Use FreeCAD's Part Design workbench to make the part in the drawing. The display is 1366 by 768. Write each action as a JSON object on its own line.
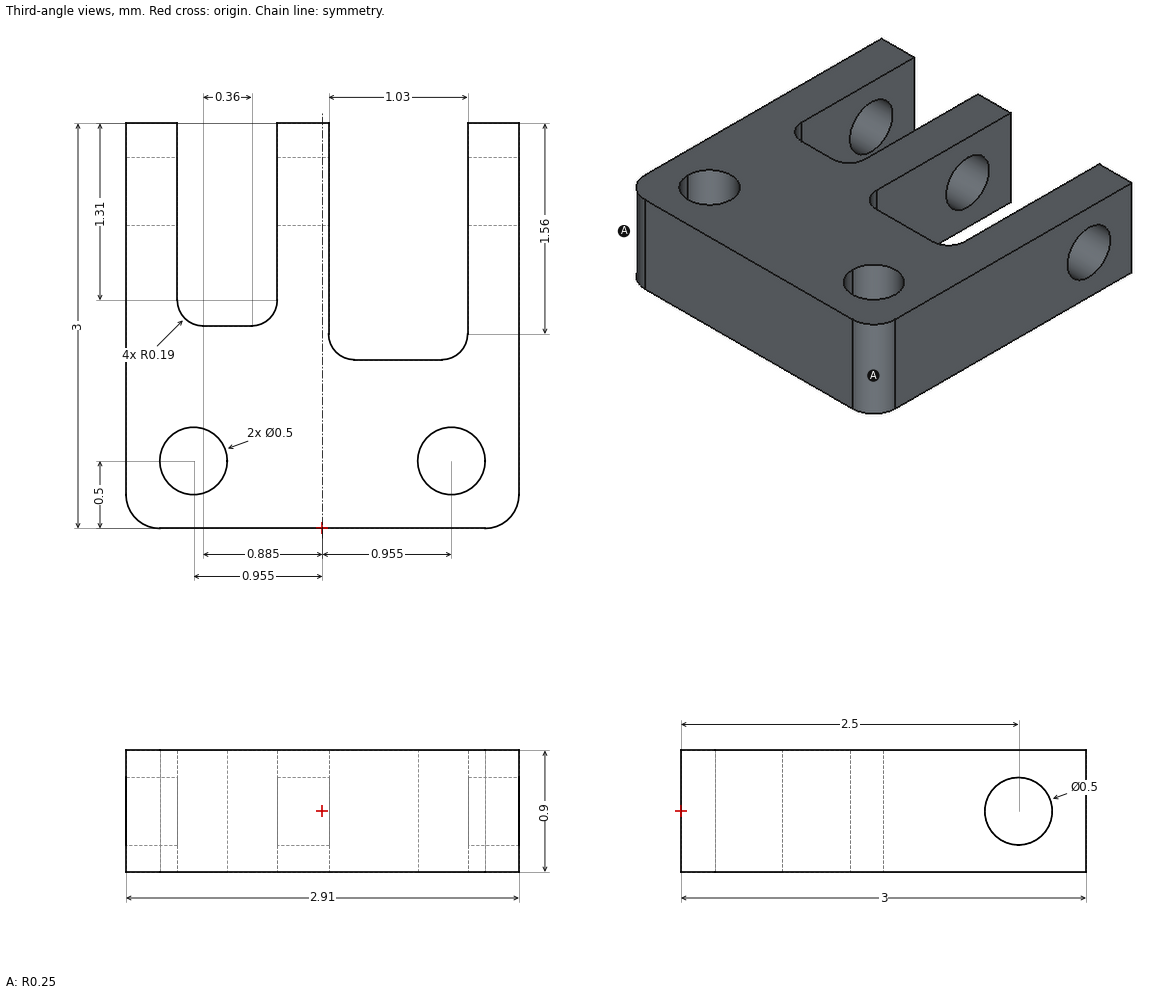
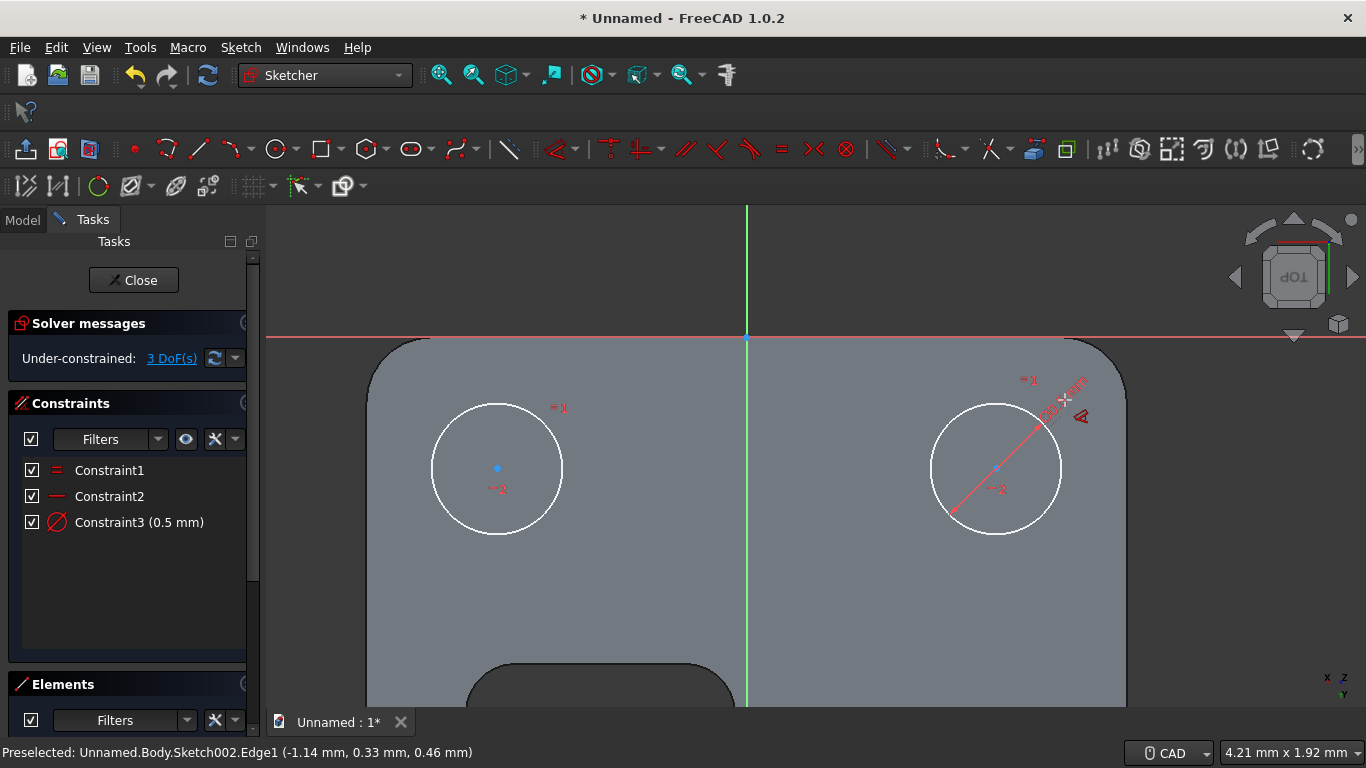
{"action": "left_click", "coordinate": [996, 469]}
{"action": "left_click", "coordinate": [1030, 373]}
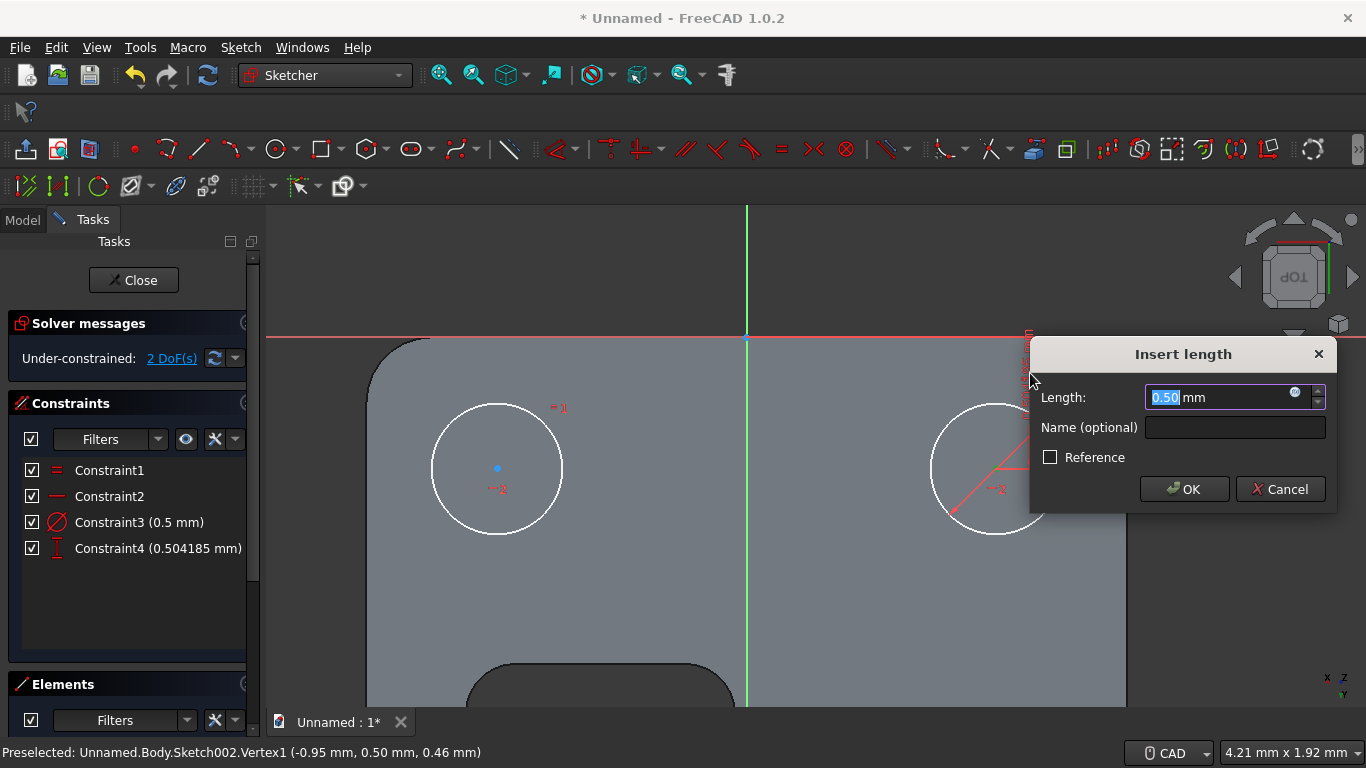
{"action": "type", "text": "0.5"}
{"action": "key", "text": "Return"}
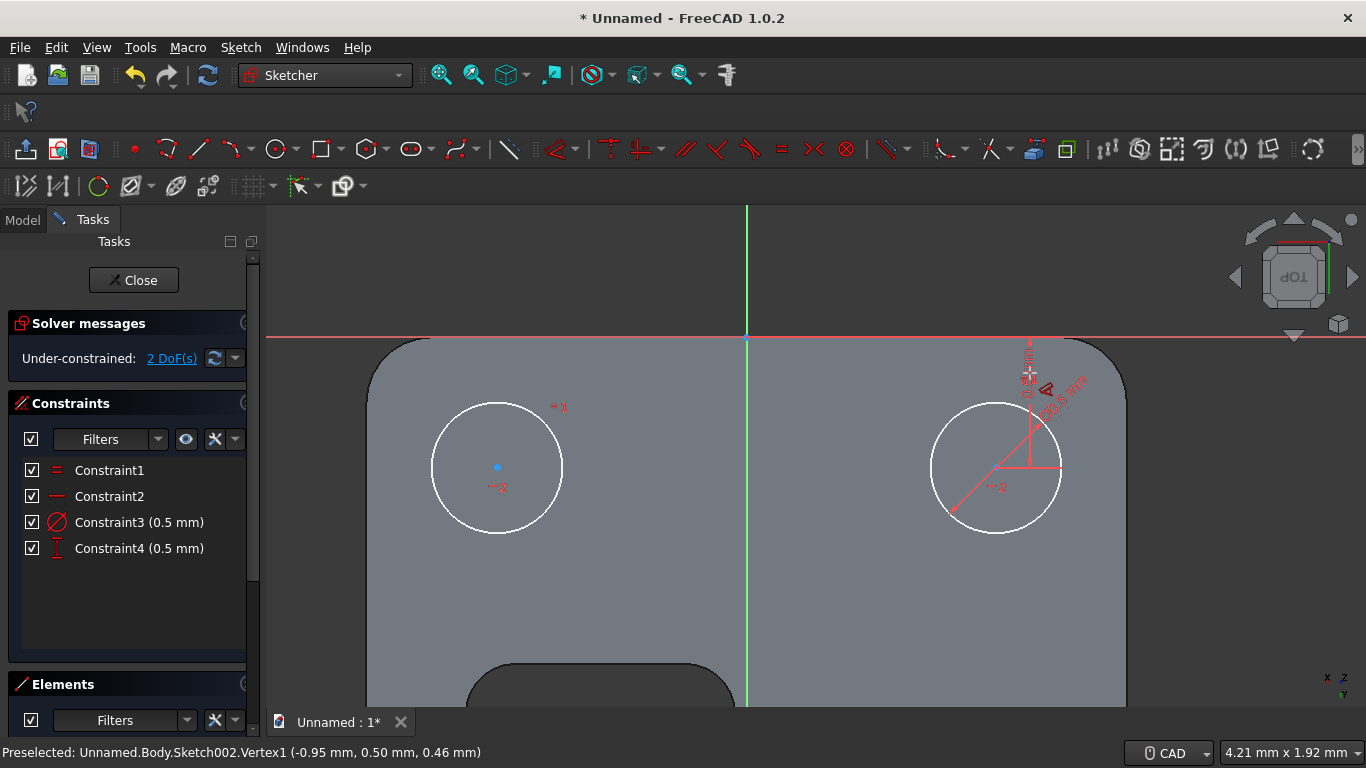
{"action": "left_click", "coordinate": [996, 468]}
{"action": "left_click", "coordinate": [871, 303]}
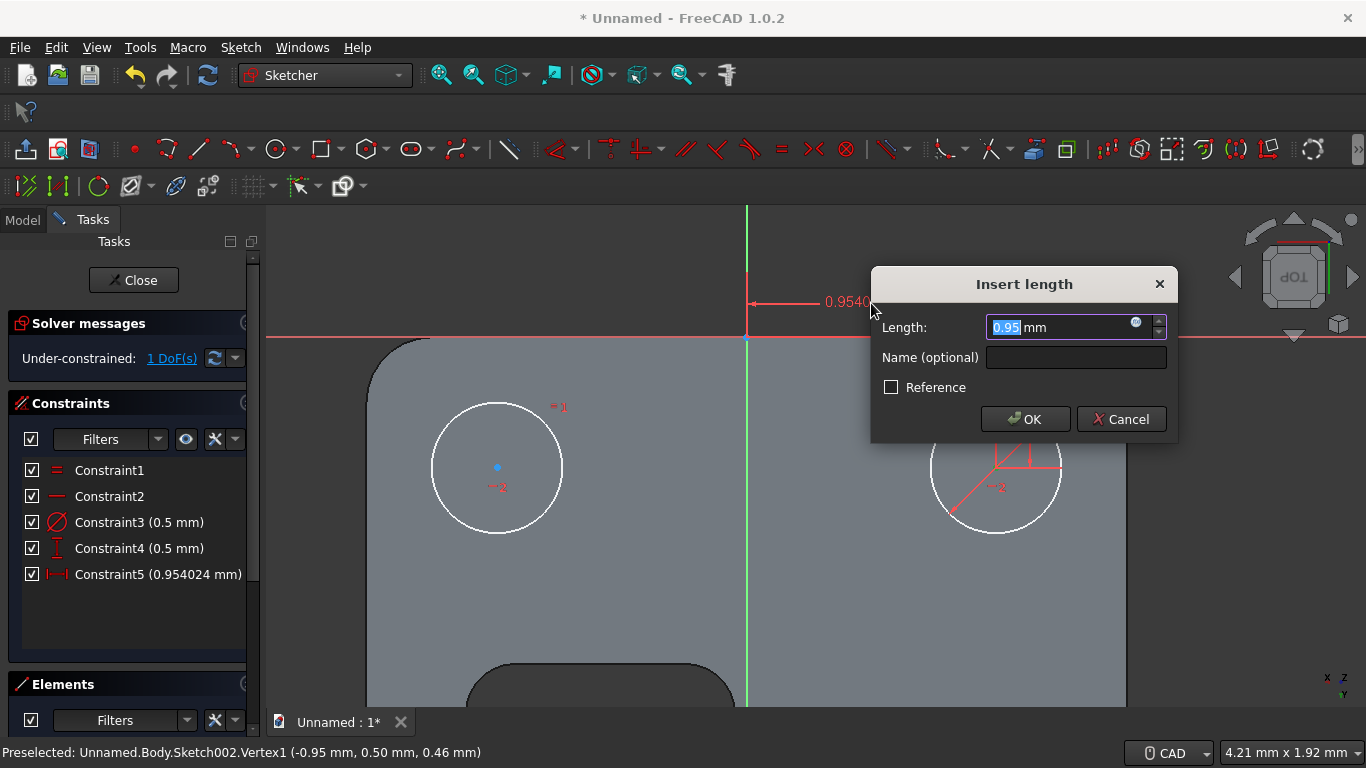
{"action": "type", "text": "0.955"}
{"action": "key", "text": "Return"}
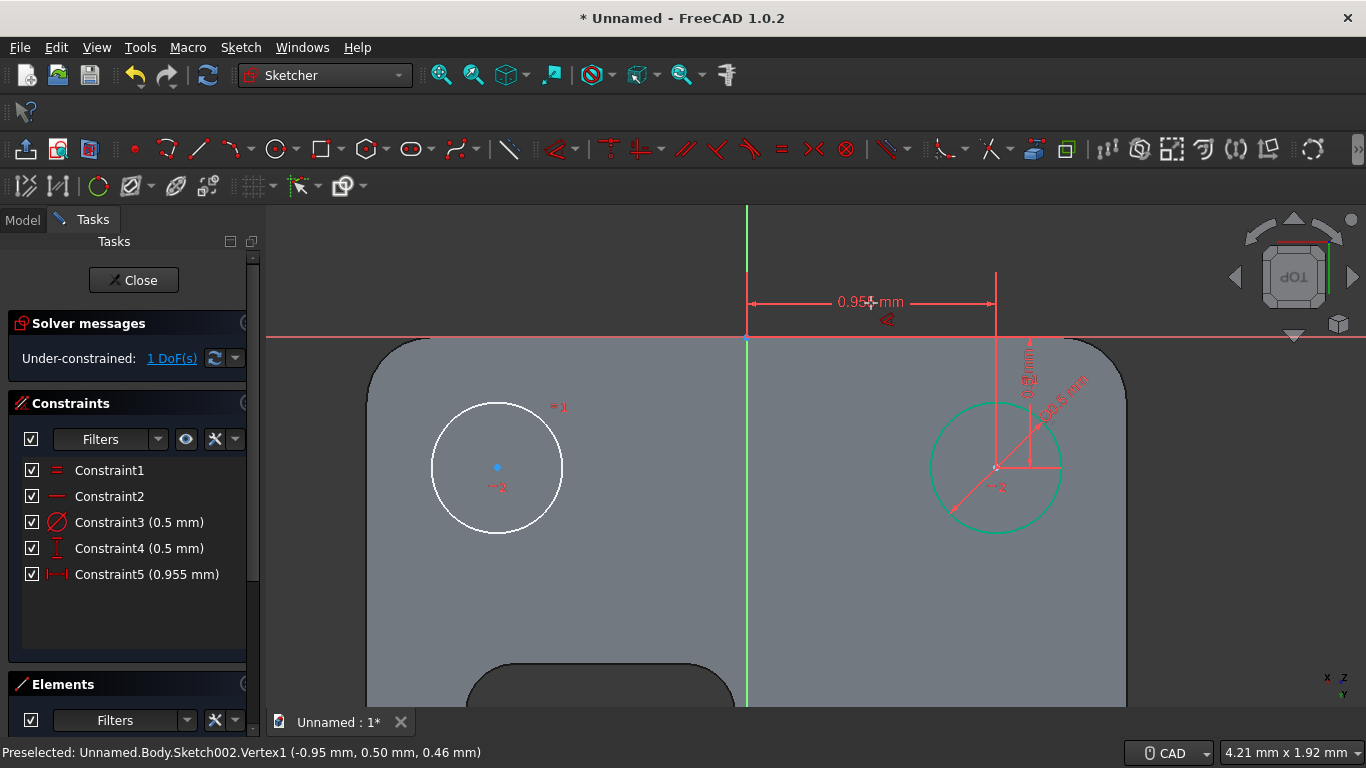
{"action": "left_click", "coordinate": [497, 468]}
{"action": "left_click", "coordinate": [622, 303]}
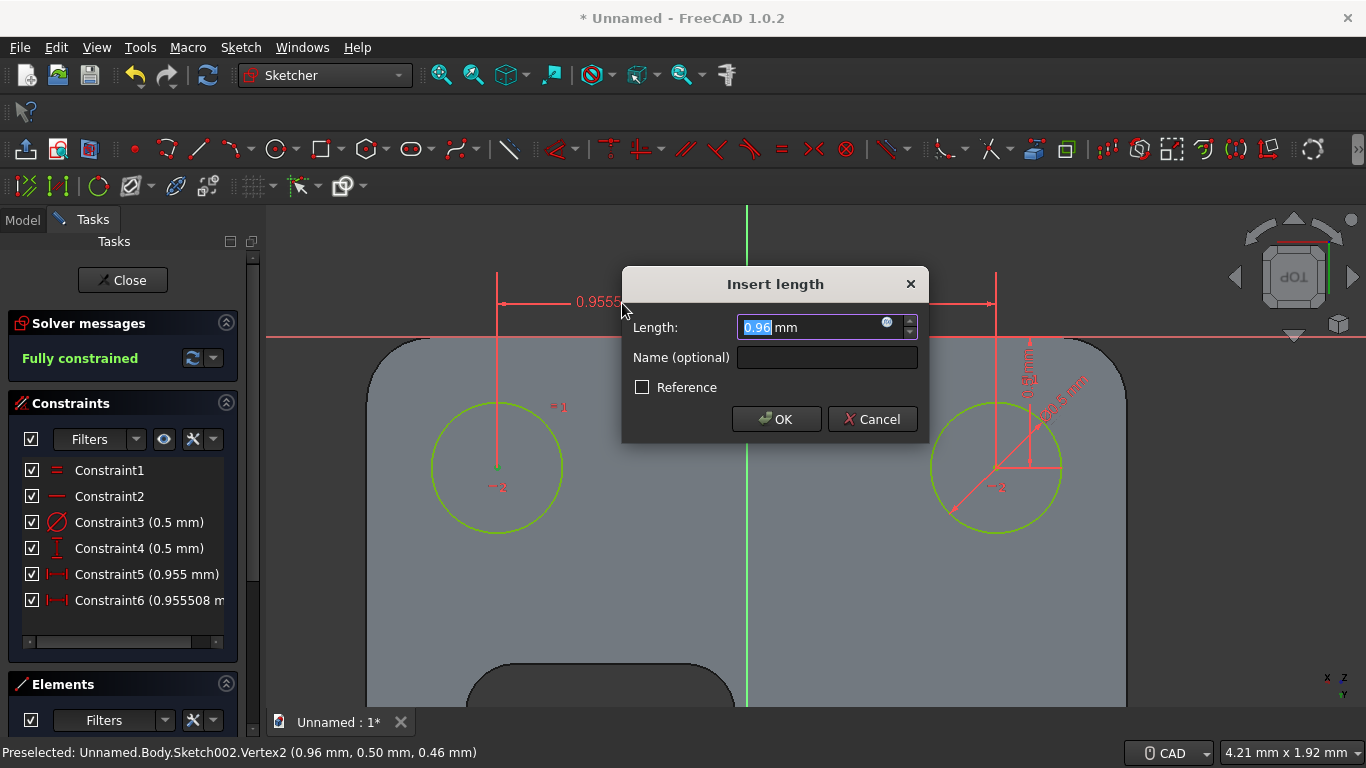
{"action": "type", "text": "0.955"}
{"action": "key", "text": "Return"}
{"action": "key", "text": "Escape"}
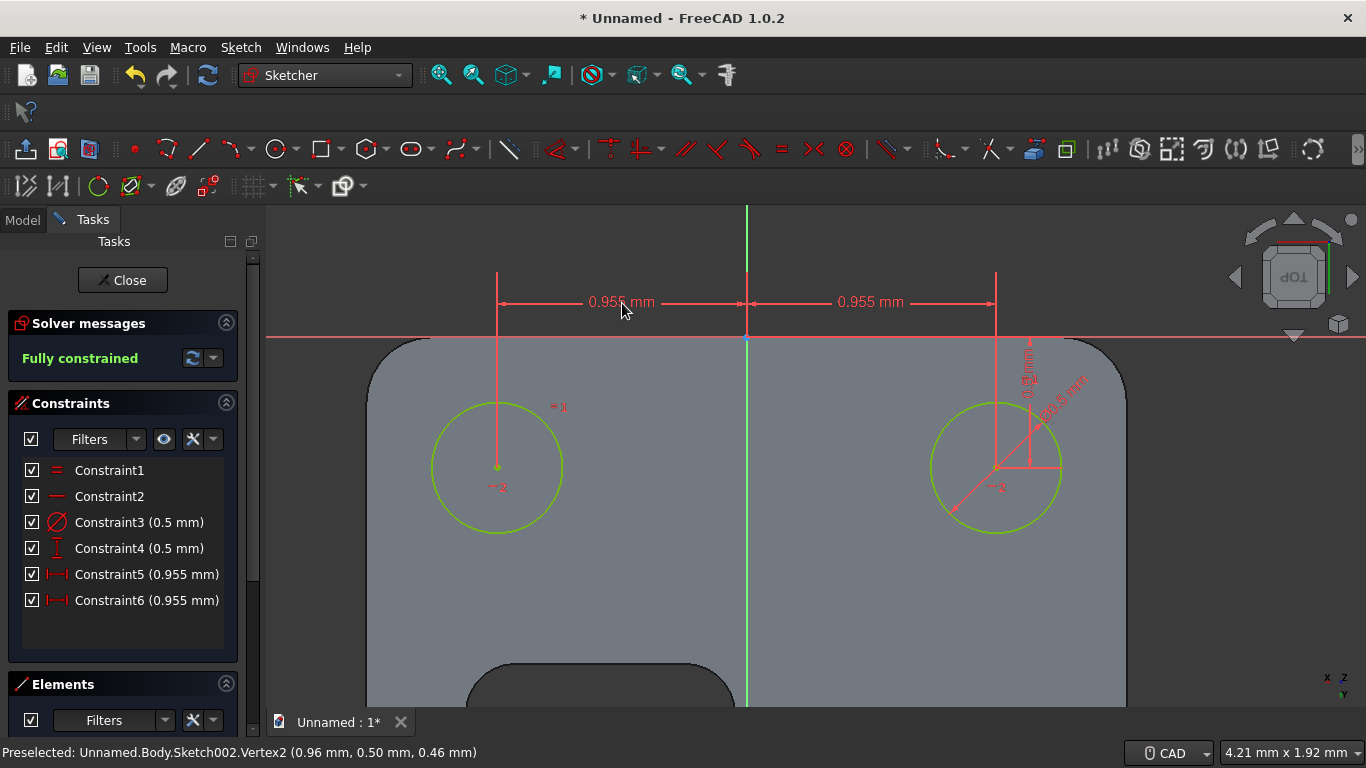
{"action": "left_click", "coordinate": [123, 280]}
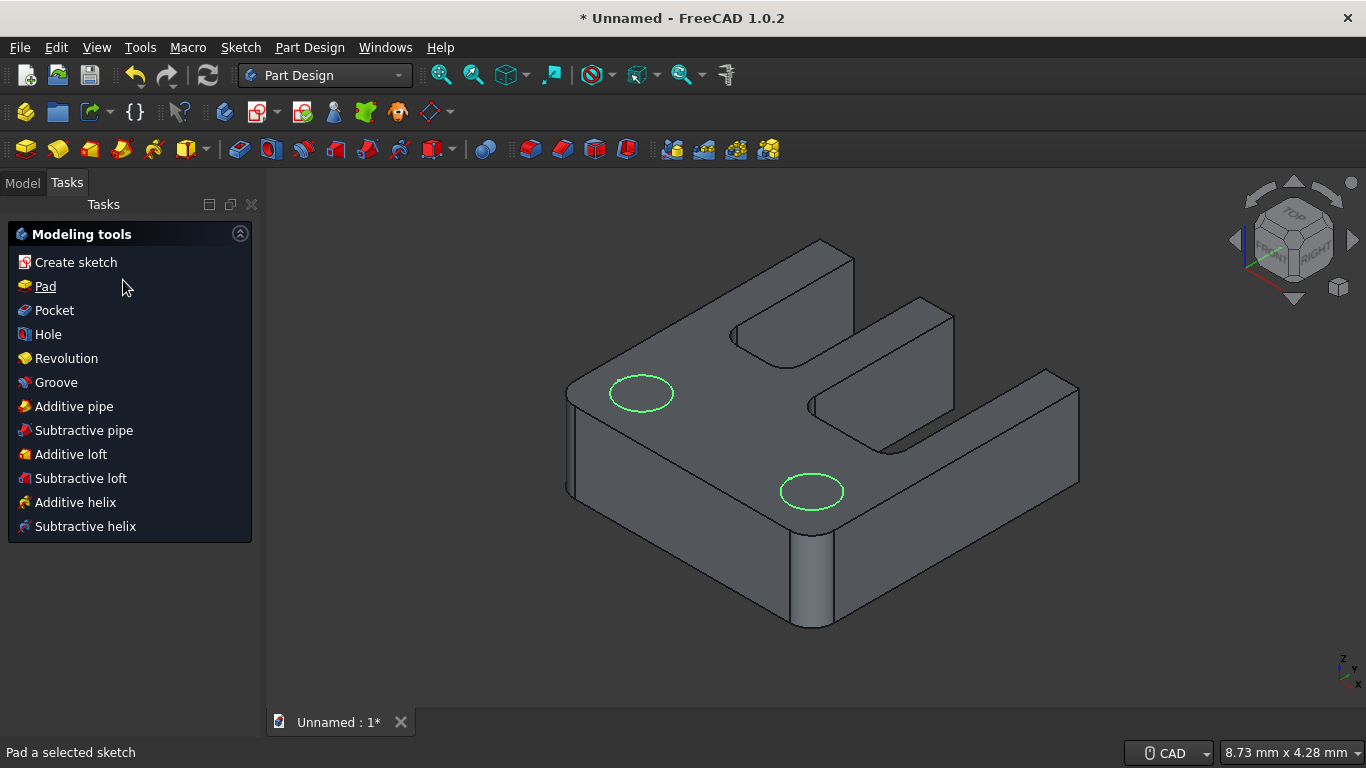
{"action": "left_click", "coordinate": [240, 150]}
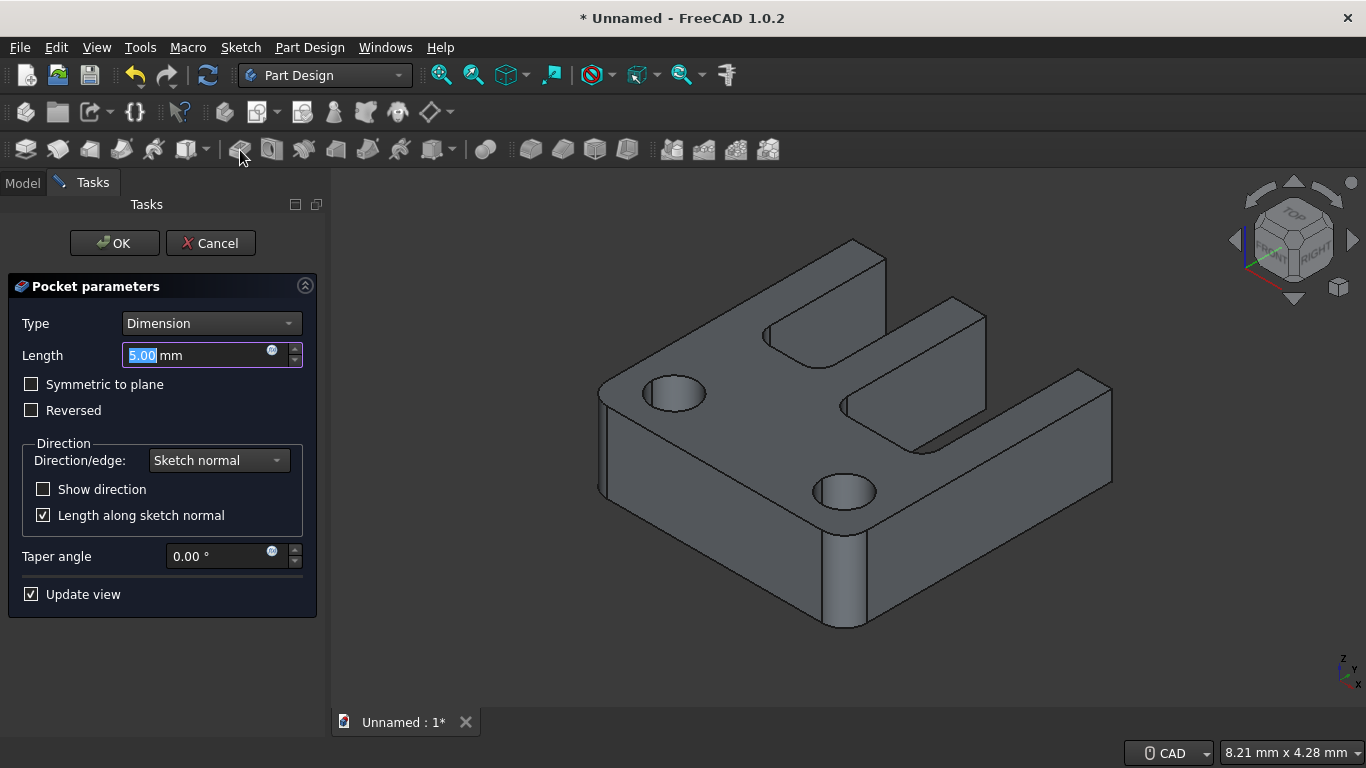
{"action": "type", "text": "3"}
{"action": "key", "text": "Tab"}